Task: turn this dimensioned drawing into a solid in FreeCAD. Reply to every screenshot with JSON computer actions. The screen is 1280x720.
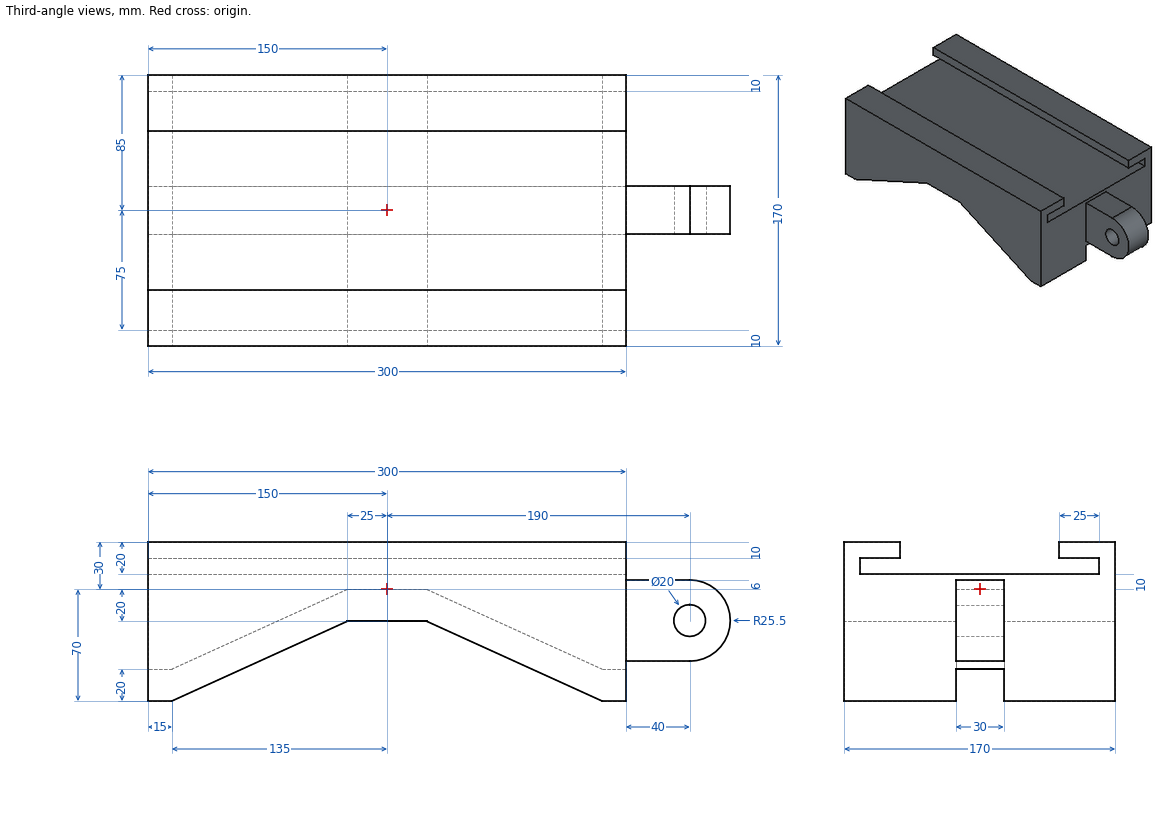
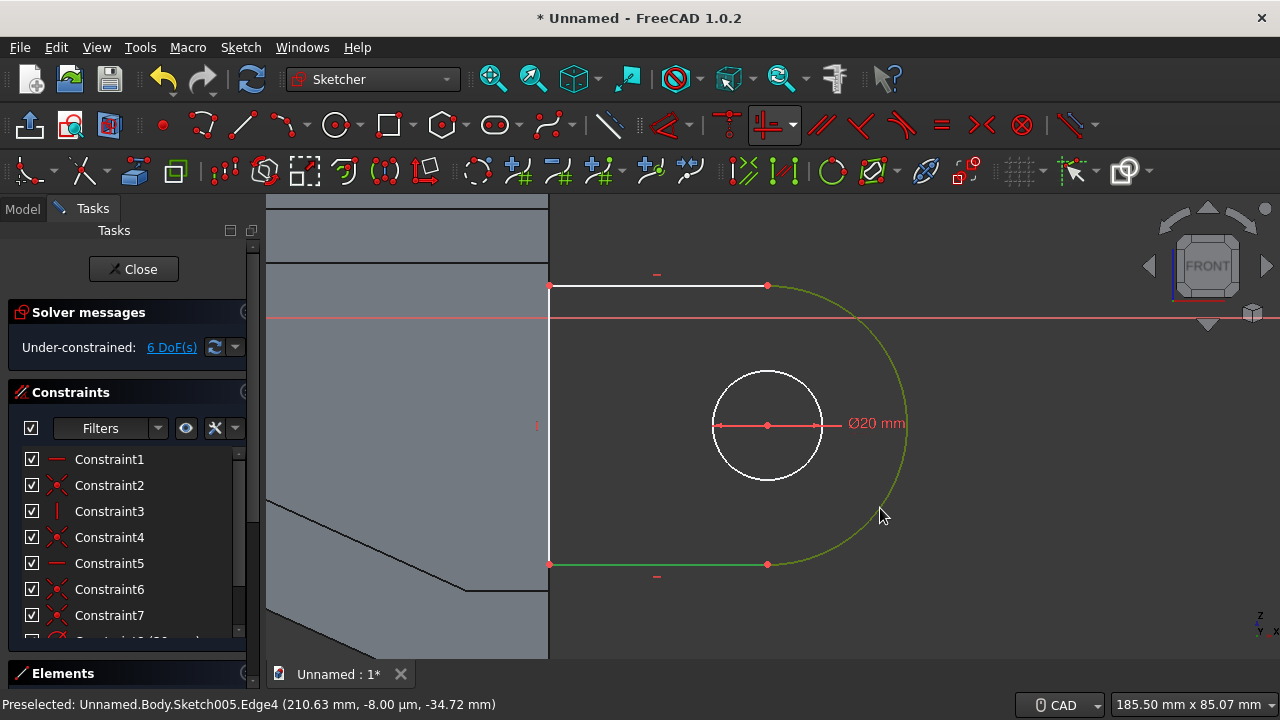
{"action": "left_click", "coordinate": [902, 126]}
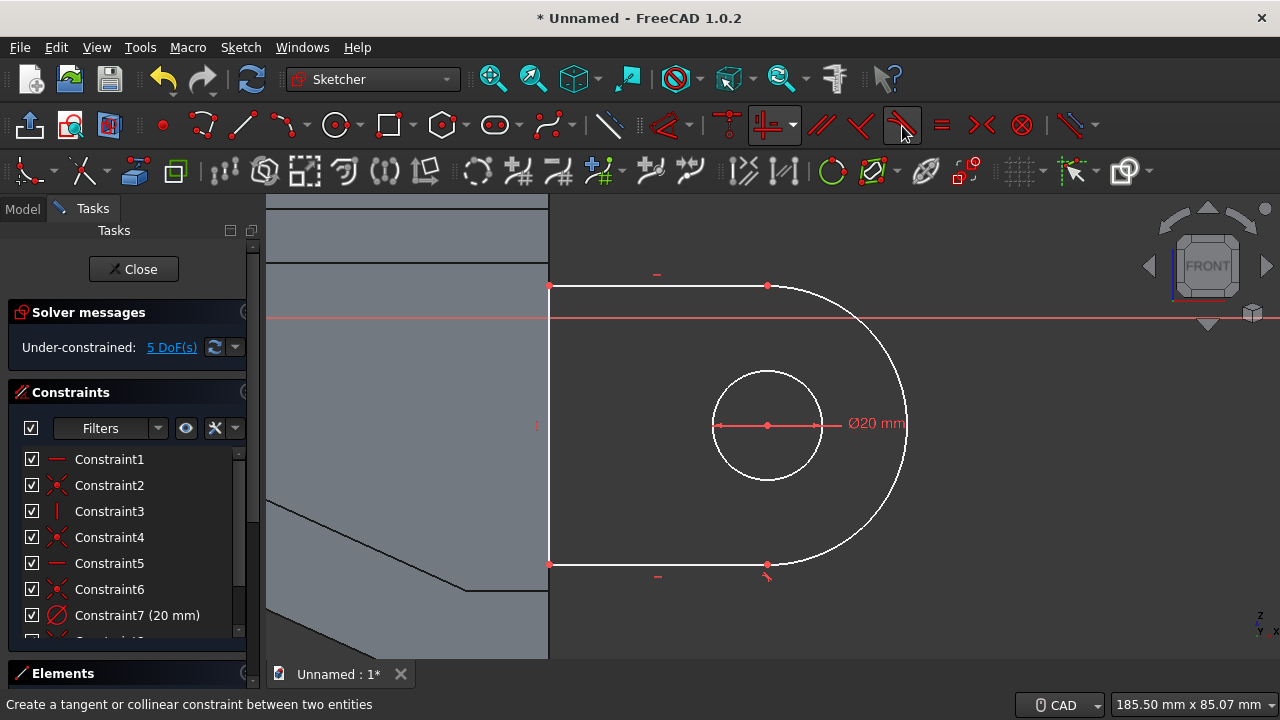
{"action": "left_click", "coordinate": [614, 286]}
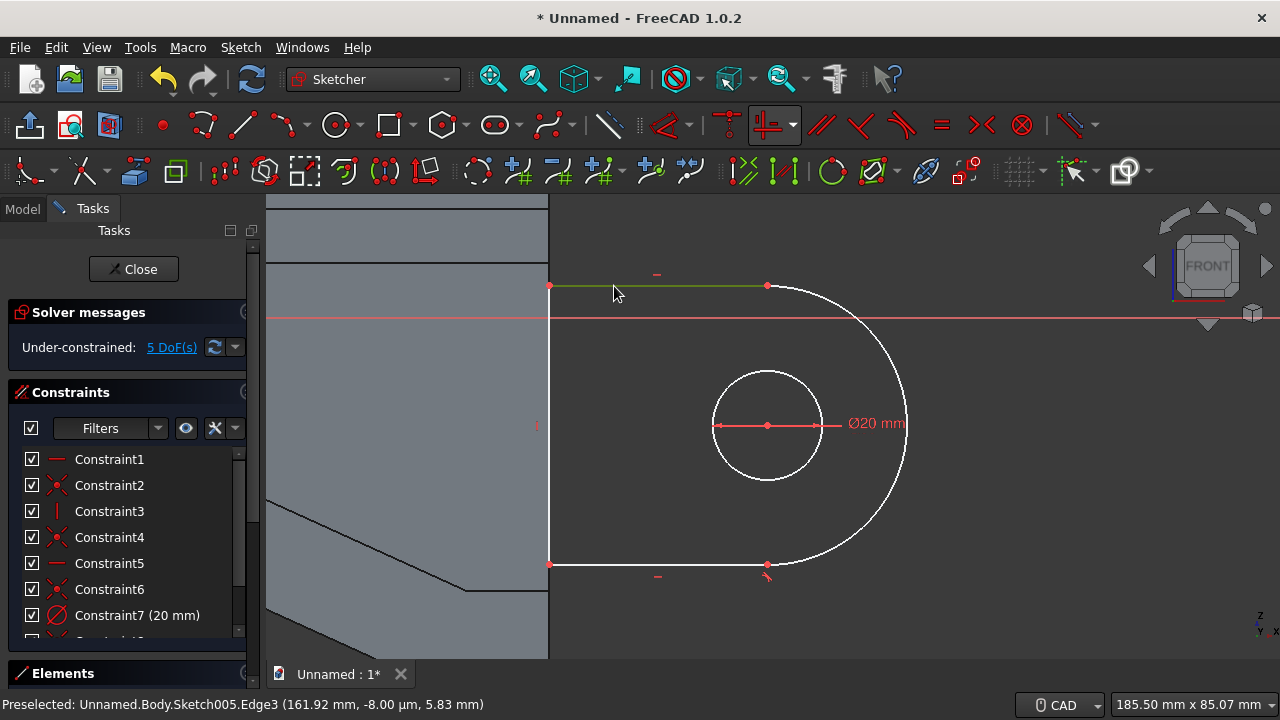
{"action": "left_click", "coordinate": [880, 507]}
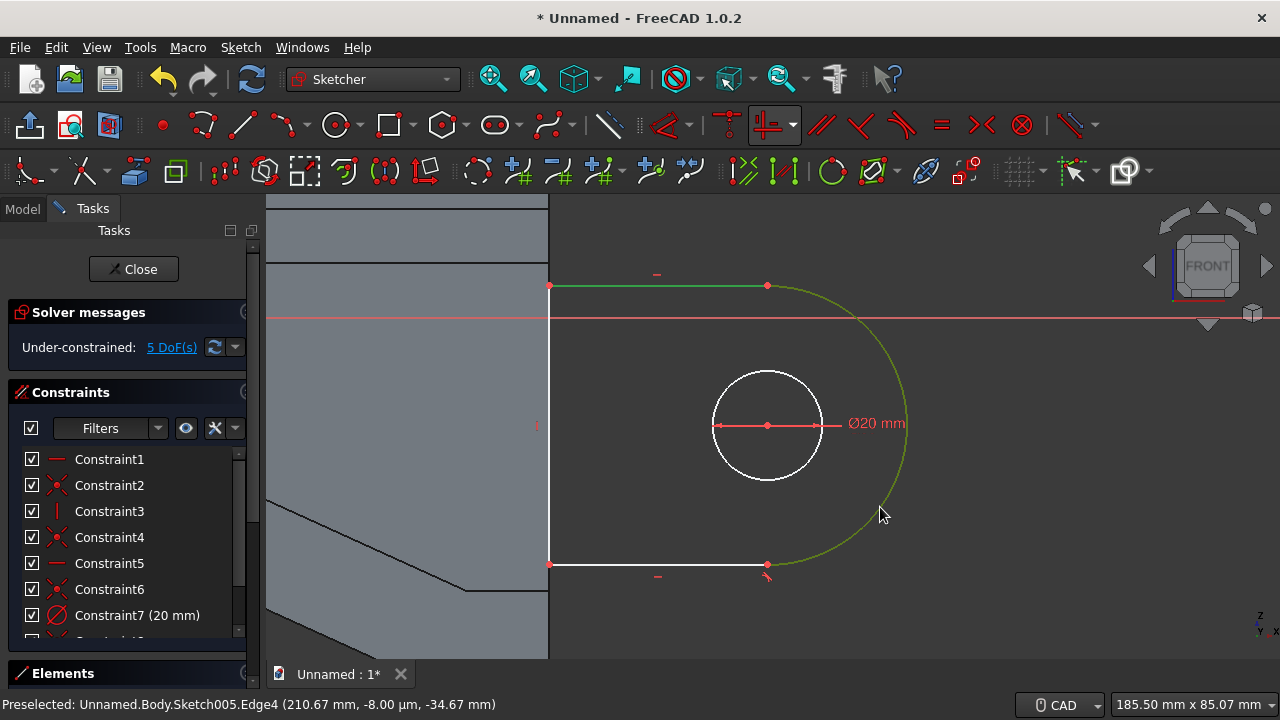
{"action": "key", "text": "t"}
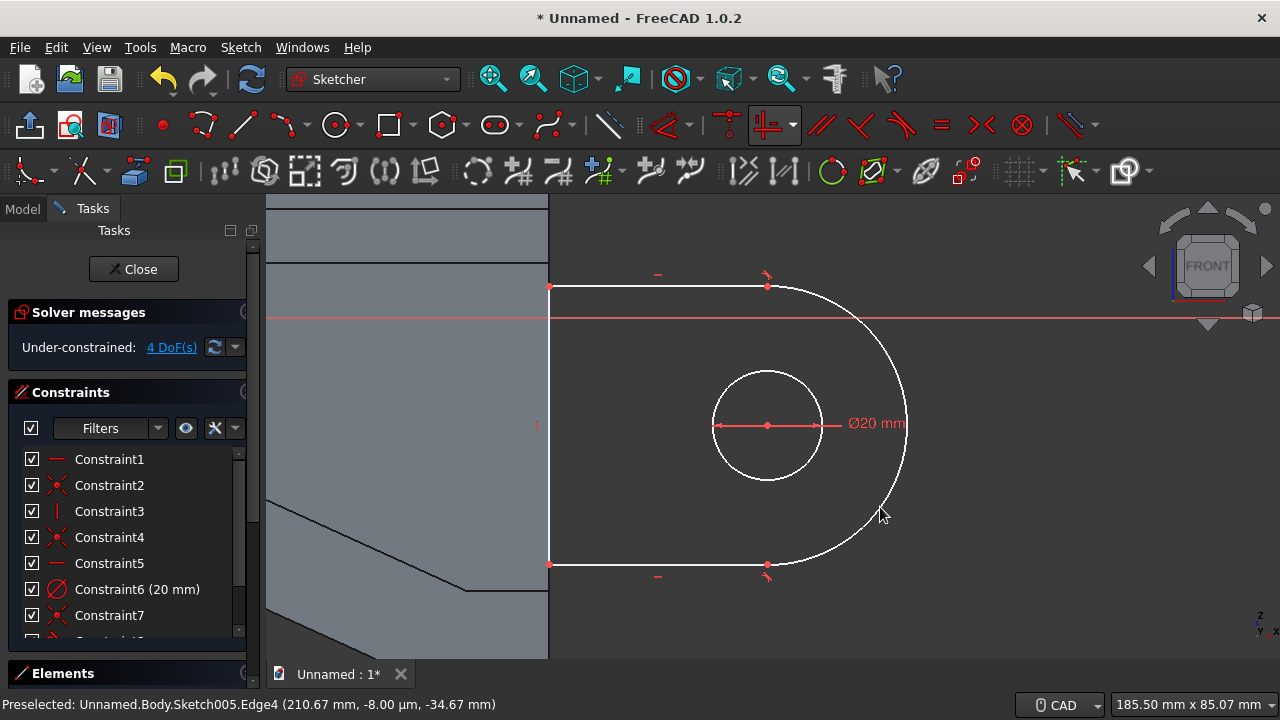
{"action": "key", "text": "d"}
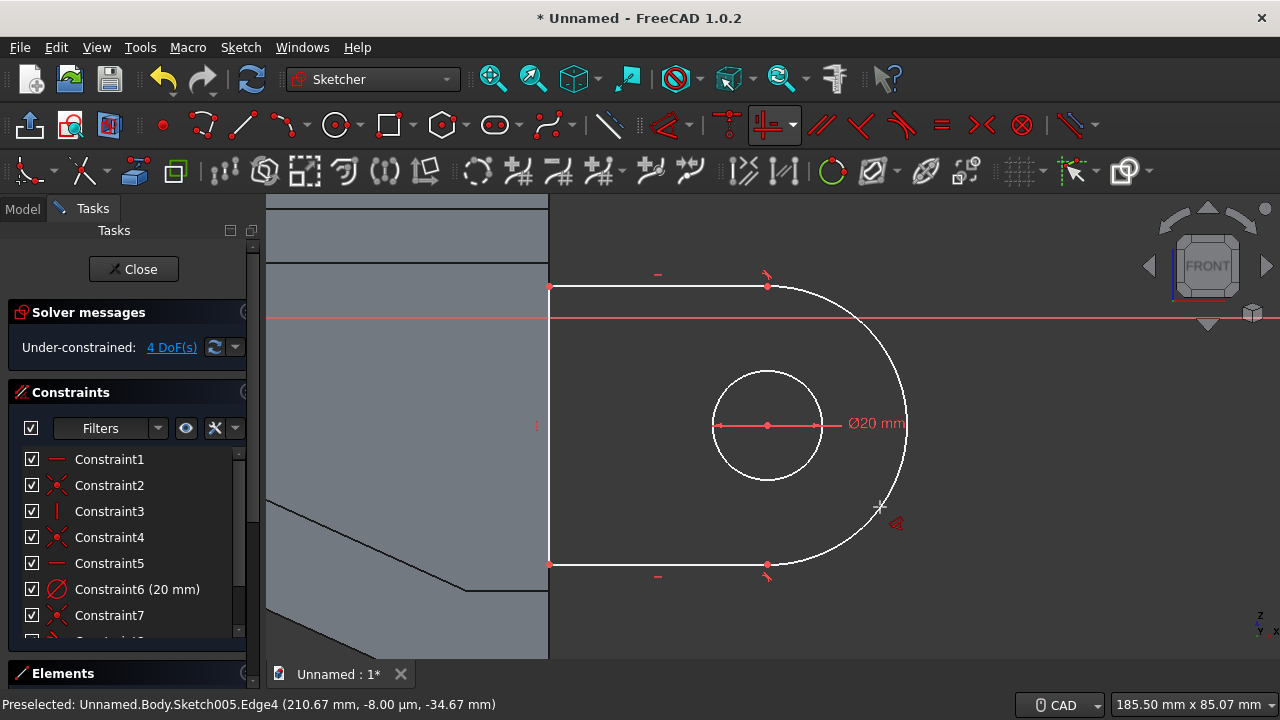
{"action": "left_click", "coordinate": [880, 507]}
{"action": "left_click", "coordinate": [906, 526]}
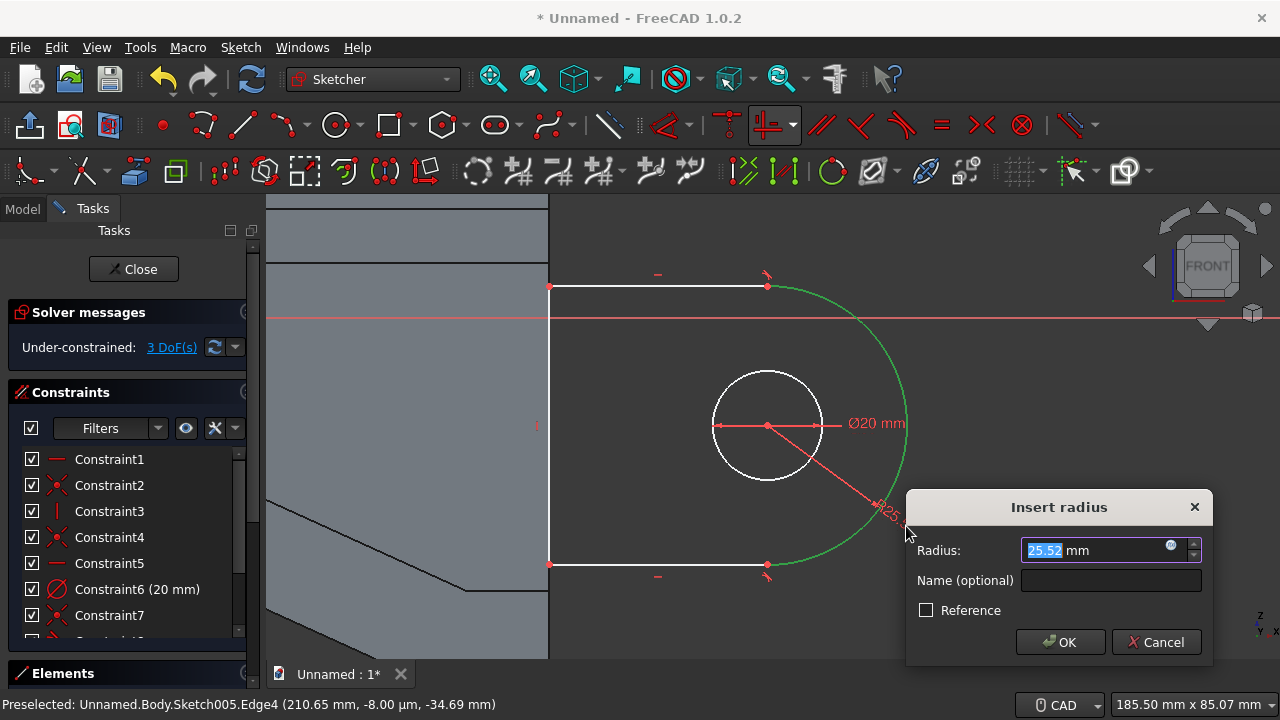
{"action": "type", "text": "25.5"}
{"action": "key", "text": "Return"}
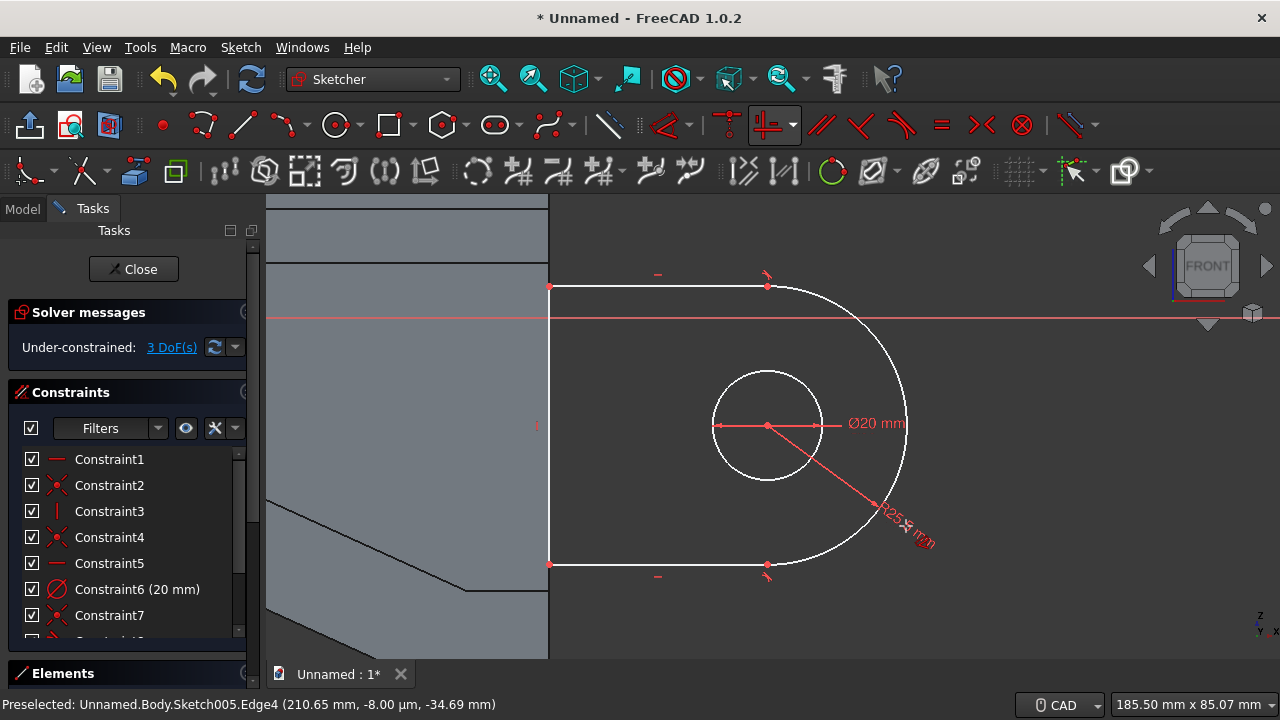
{"action": "left_click", "coordinate": [702, 565]}
{"action": "left_click", "coordinate": [658, 599]}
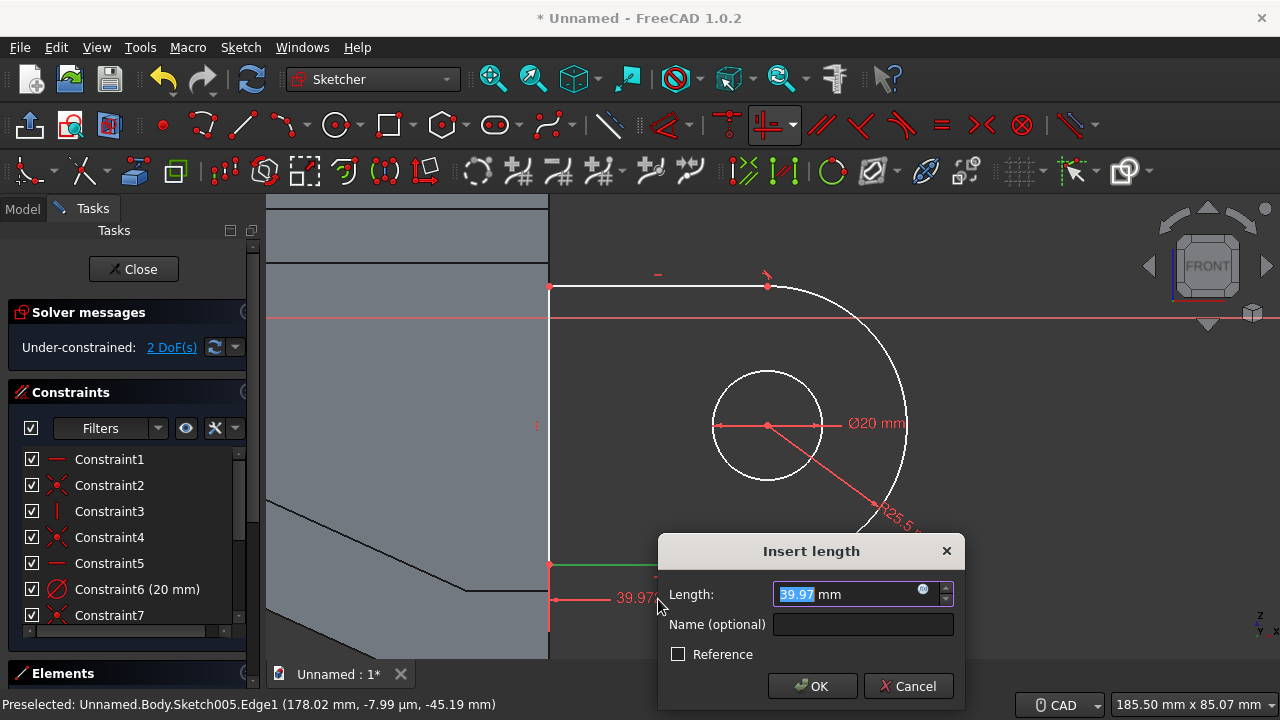
{"action": "type", "text": "40"}
{"action": "key", "text": "Return"}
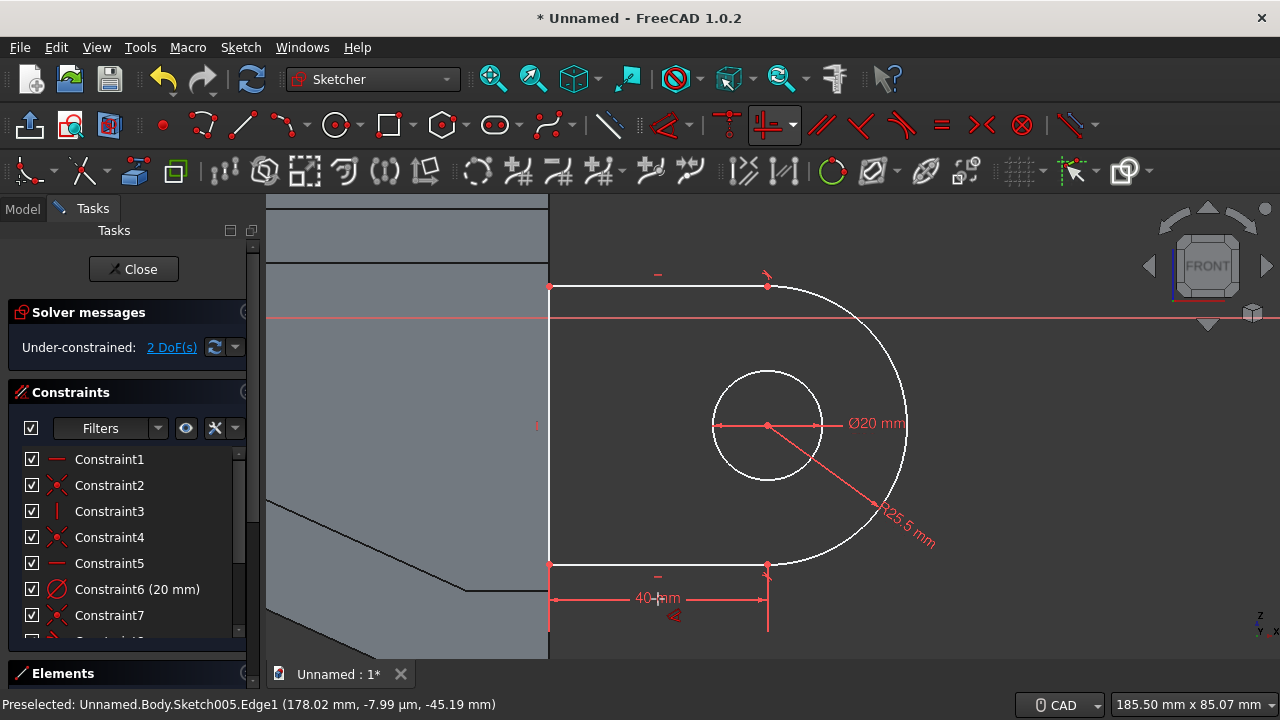
{"action": "left_click", "coordinate": [549, 286]}
{"action": "left_click", "coordinate": [583, 302]}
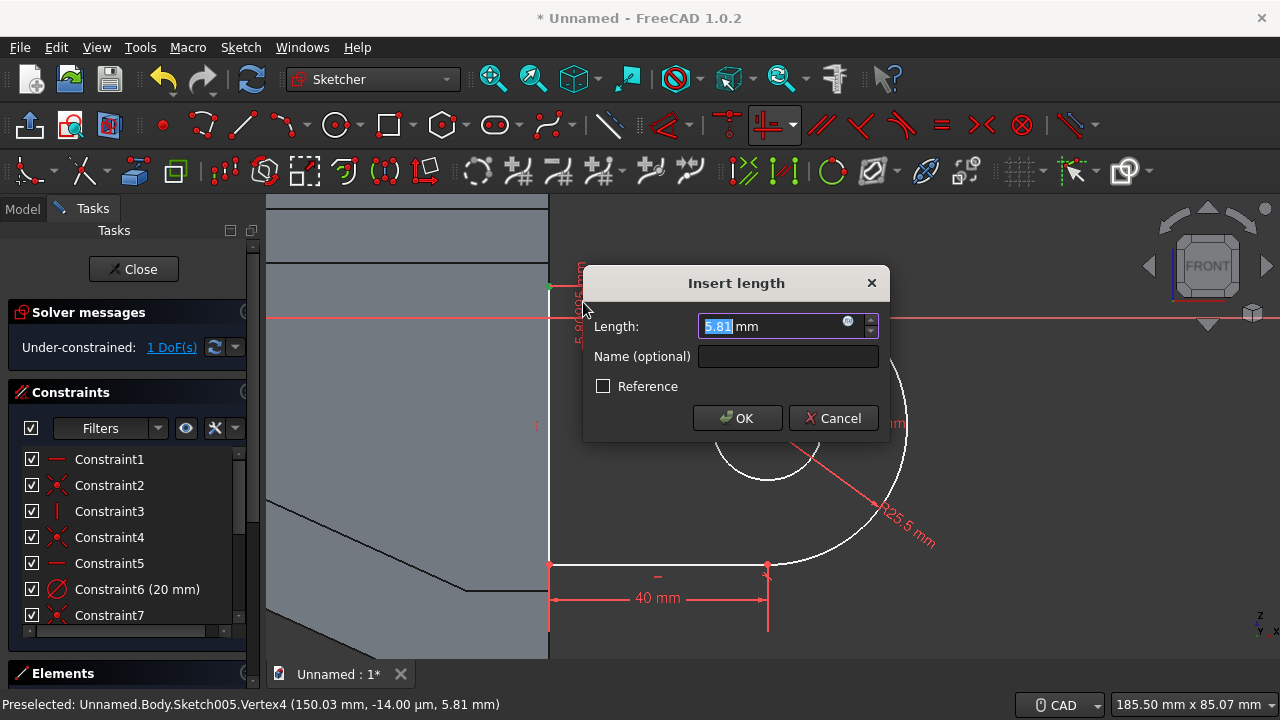
{"action": "type", "text": "6"}
{"action": "key", "text": "Return"}